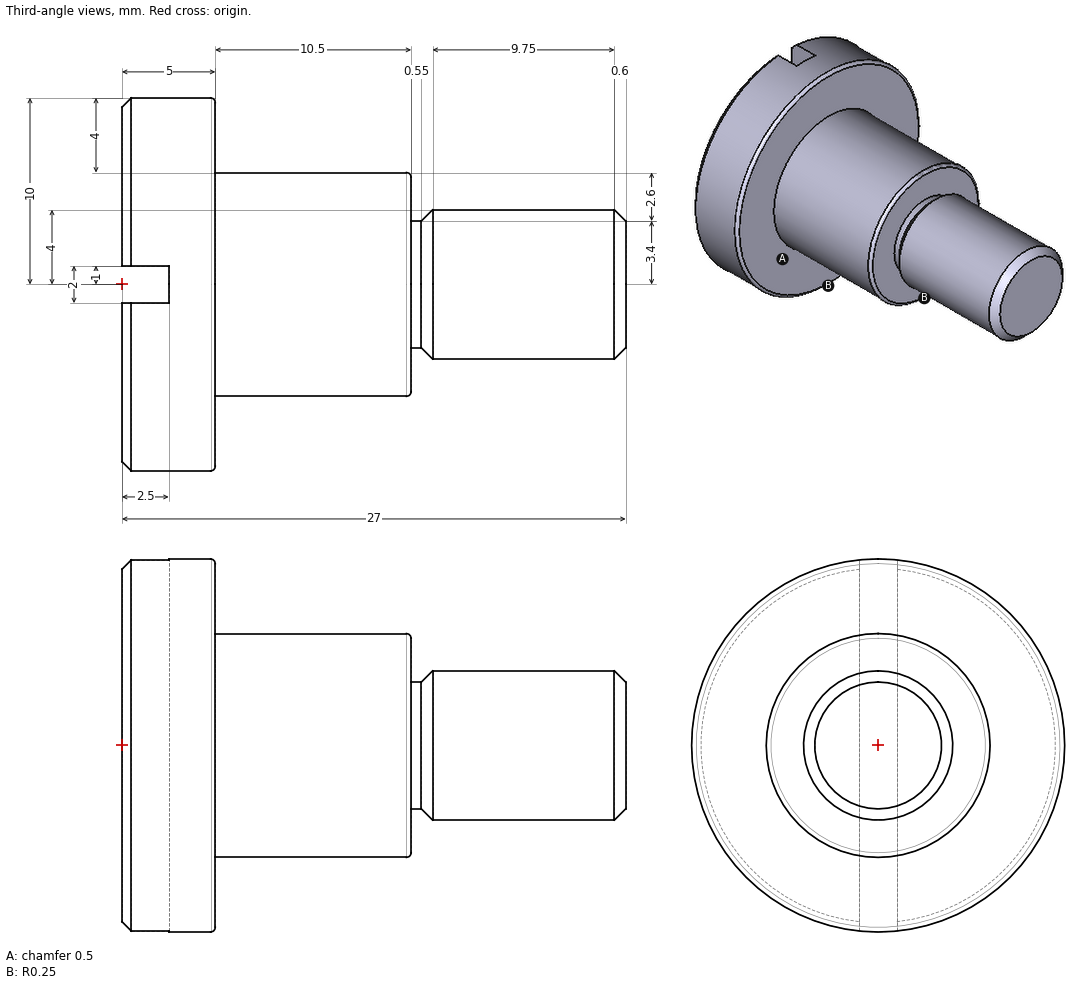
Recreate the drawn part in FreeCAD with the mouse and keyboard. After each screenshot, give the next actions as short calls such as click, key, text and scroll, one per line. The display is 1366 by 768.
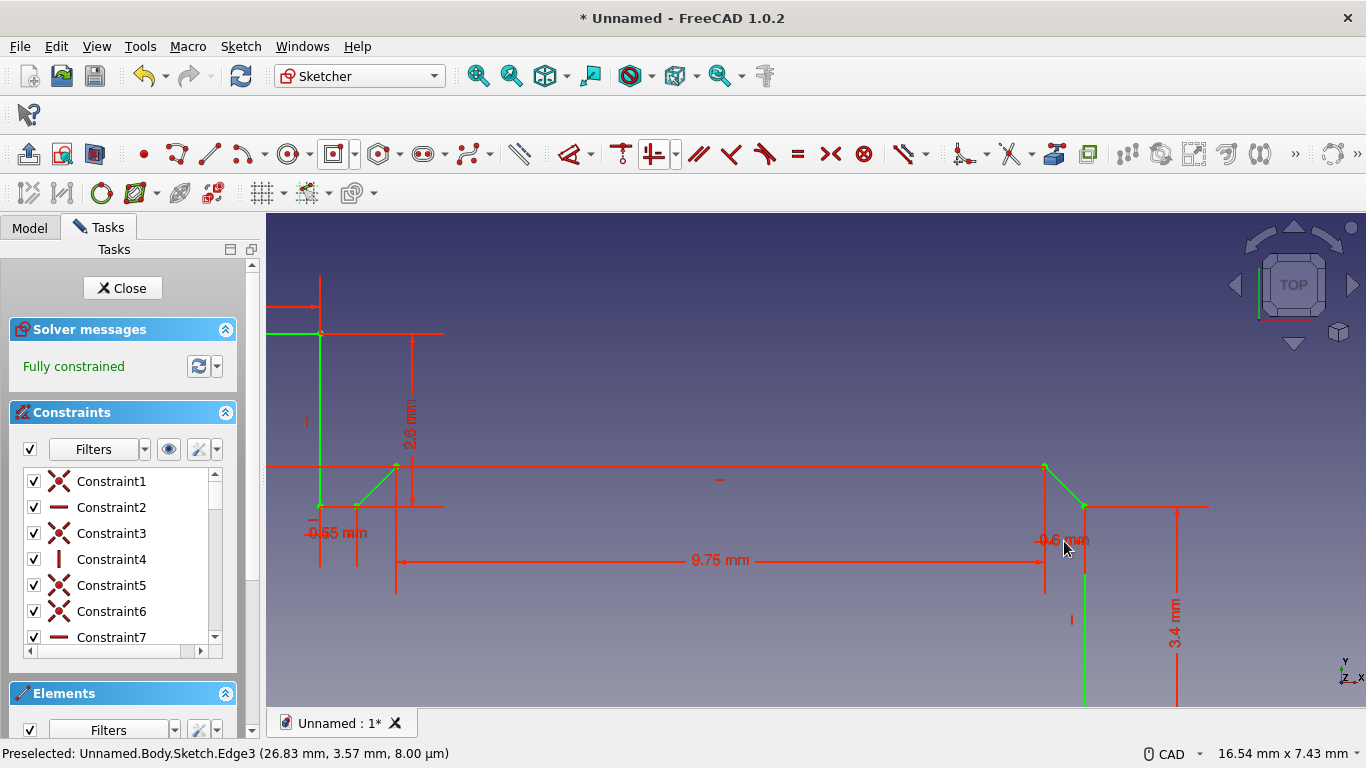
click(123, 288)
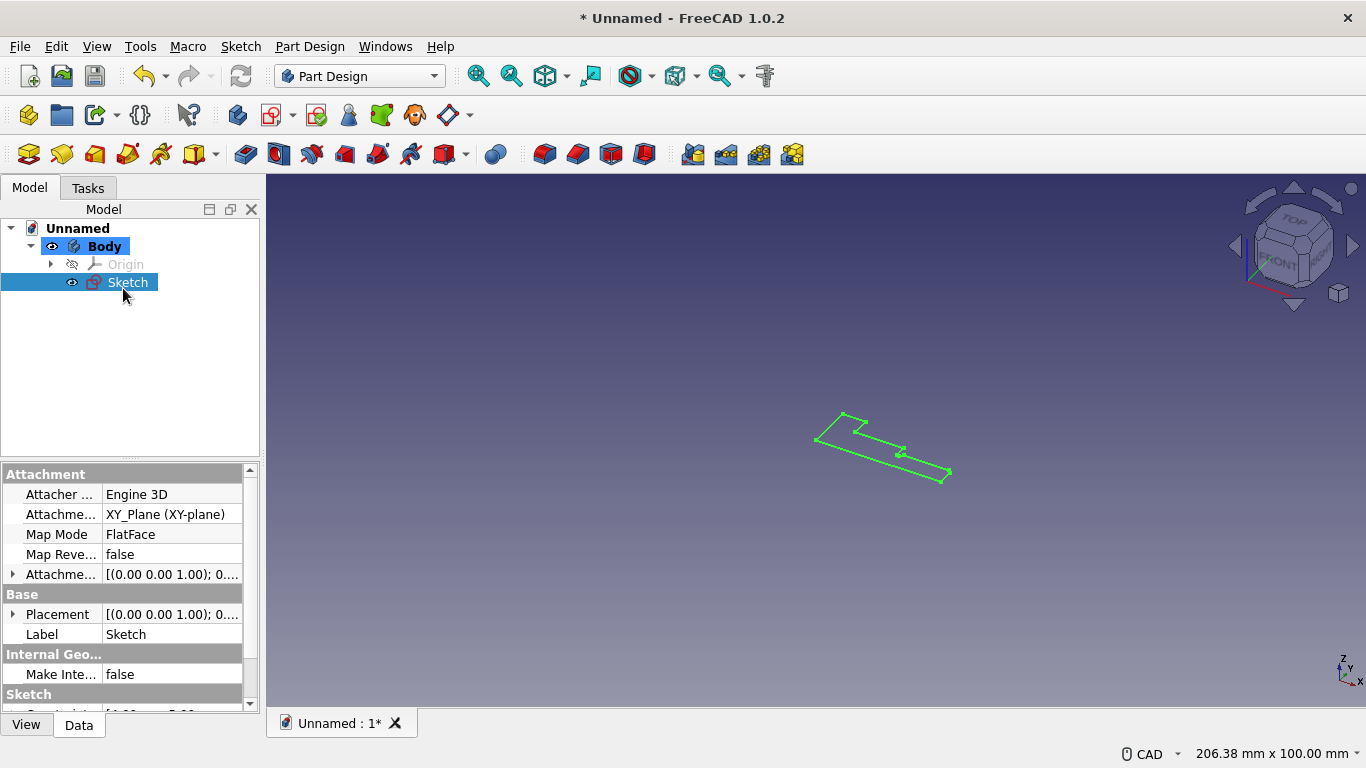
click(62, 154)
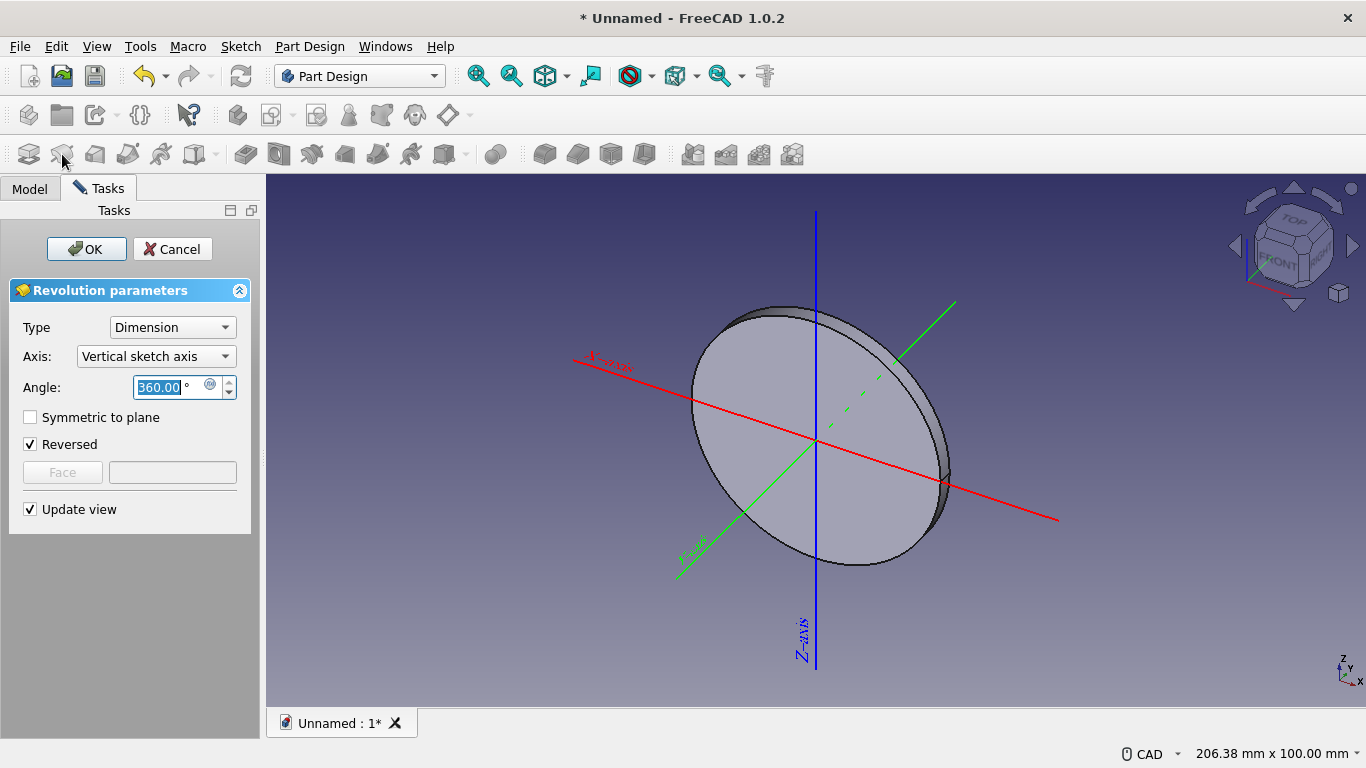
click(157, 356)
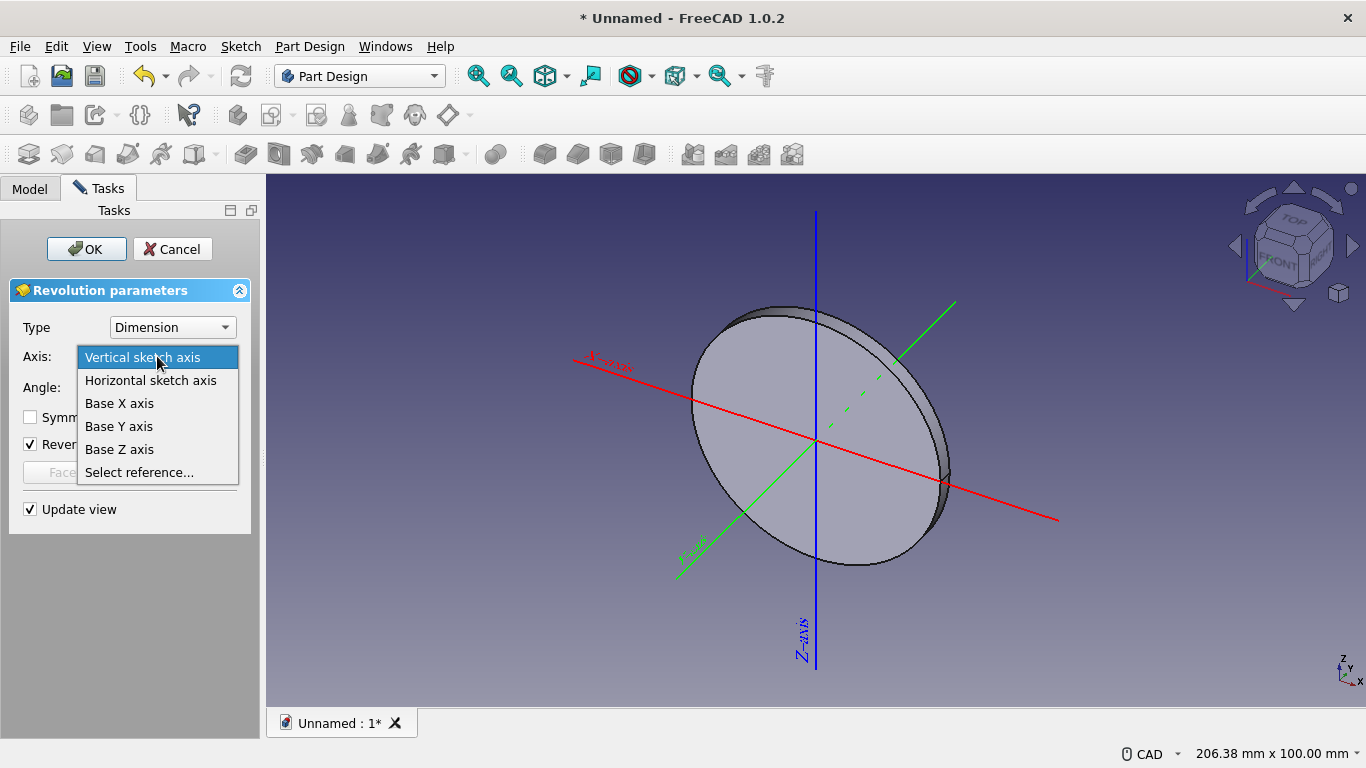
click(156, 380)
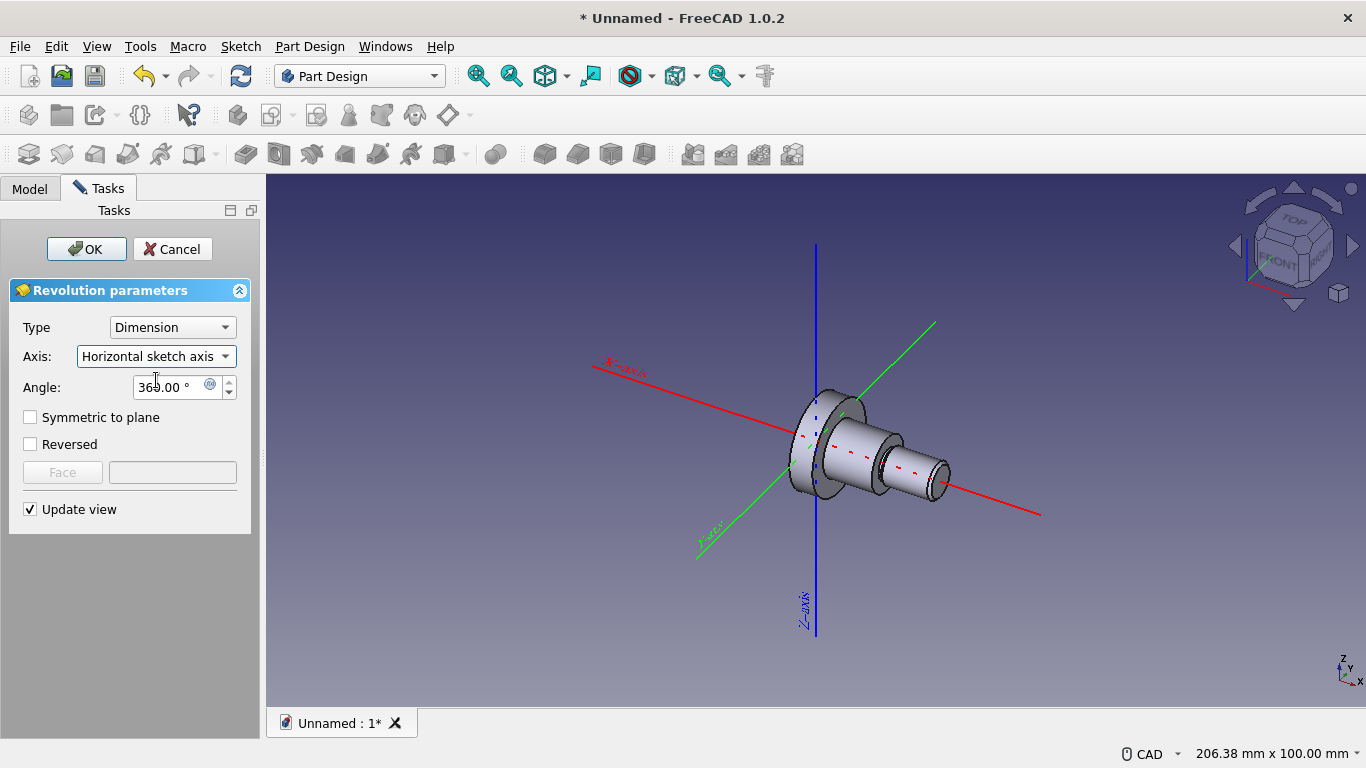
click(87, 249)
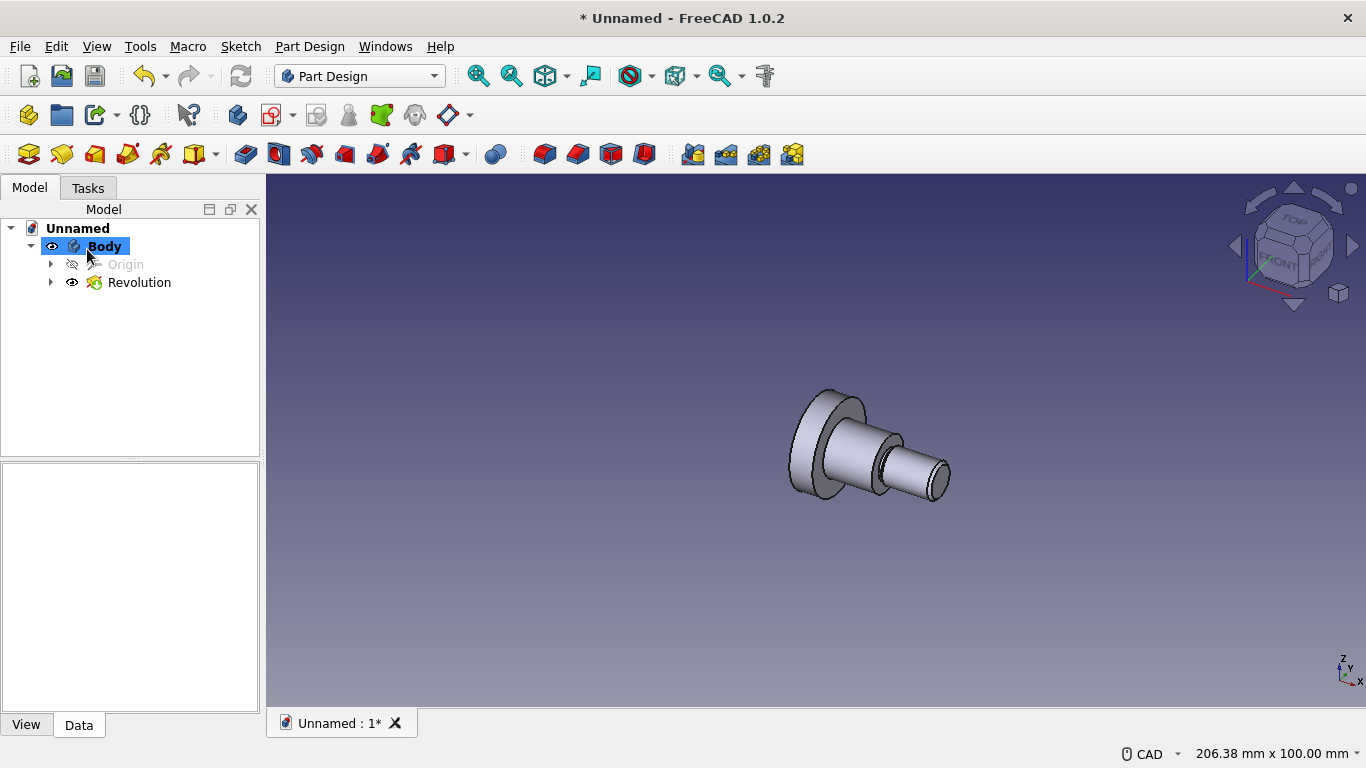
click(479, 76)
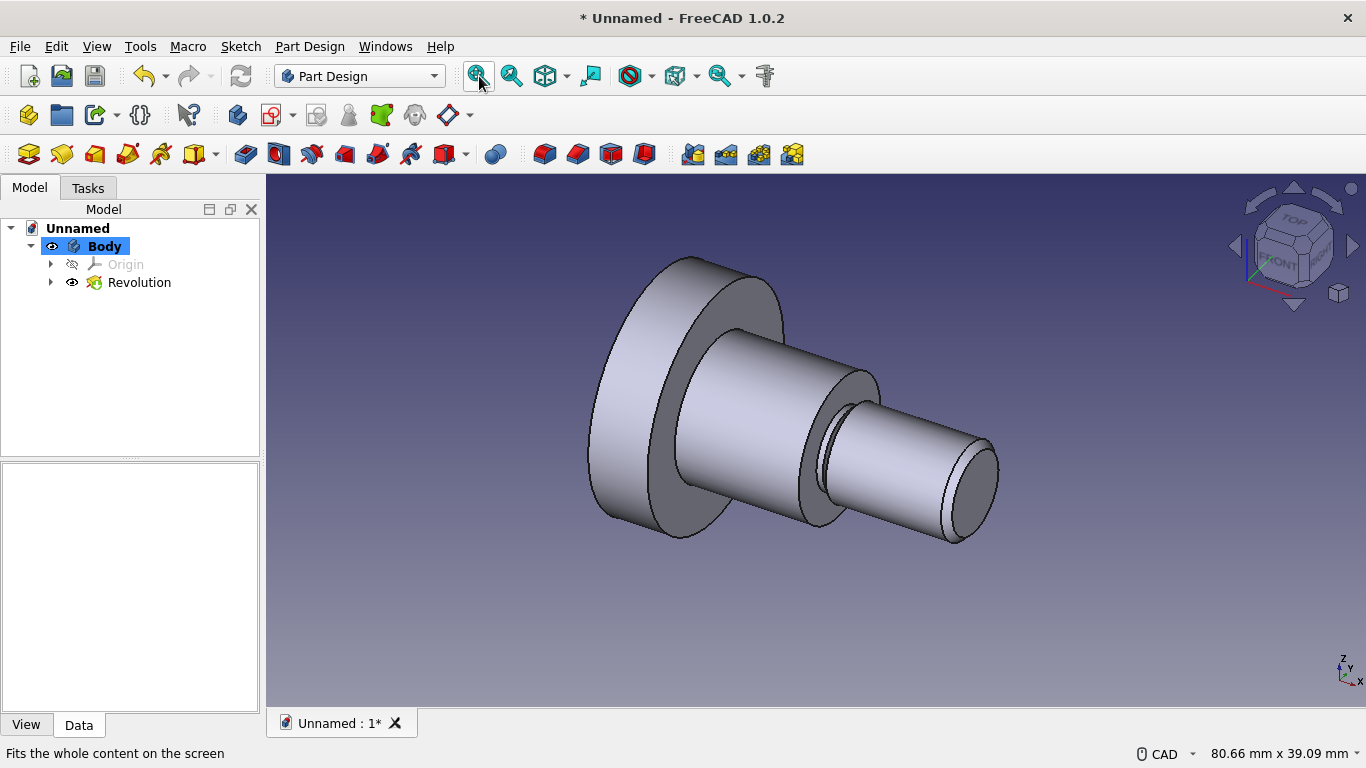
key(0)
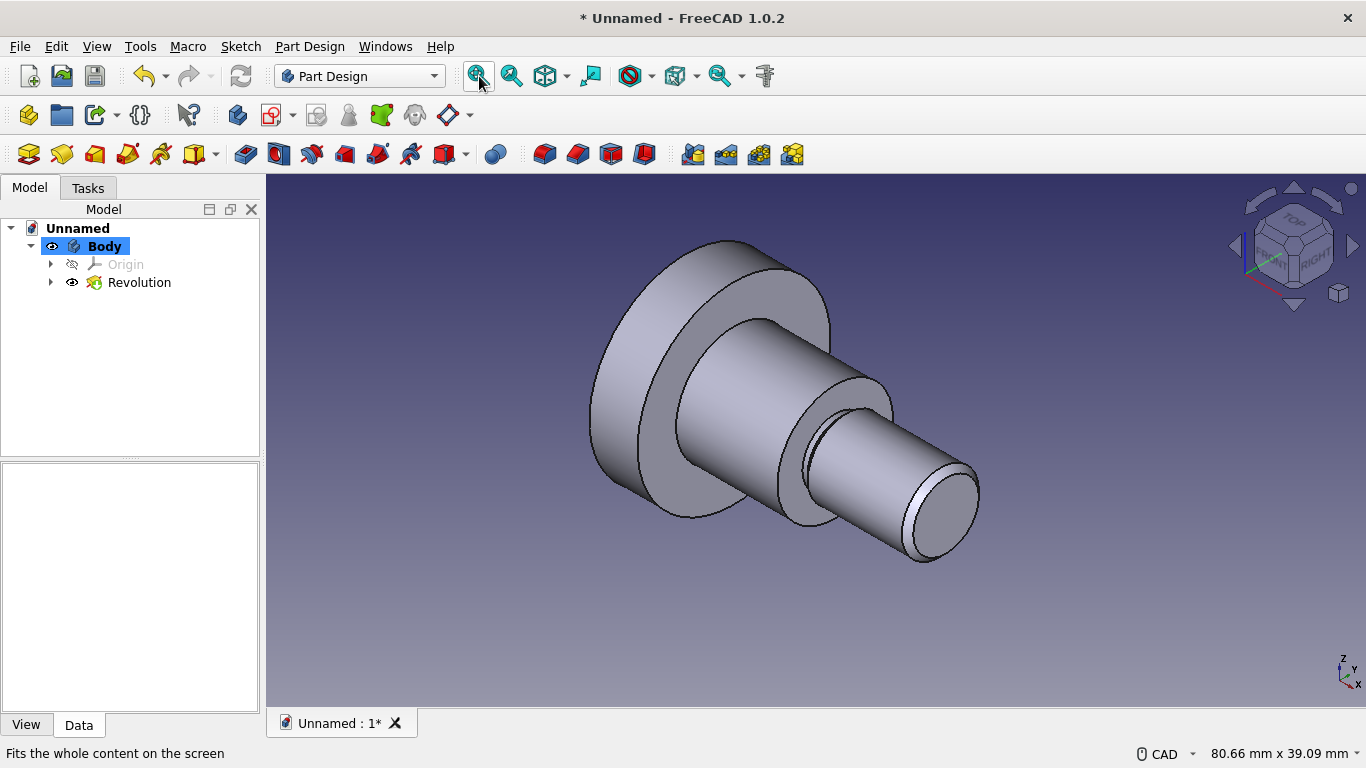
key(2)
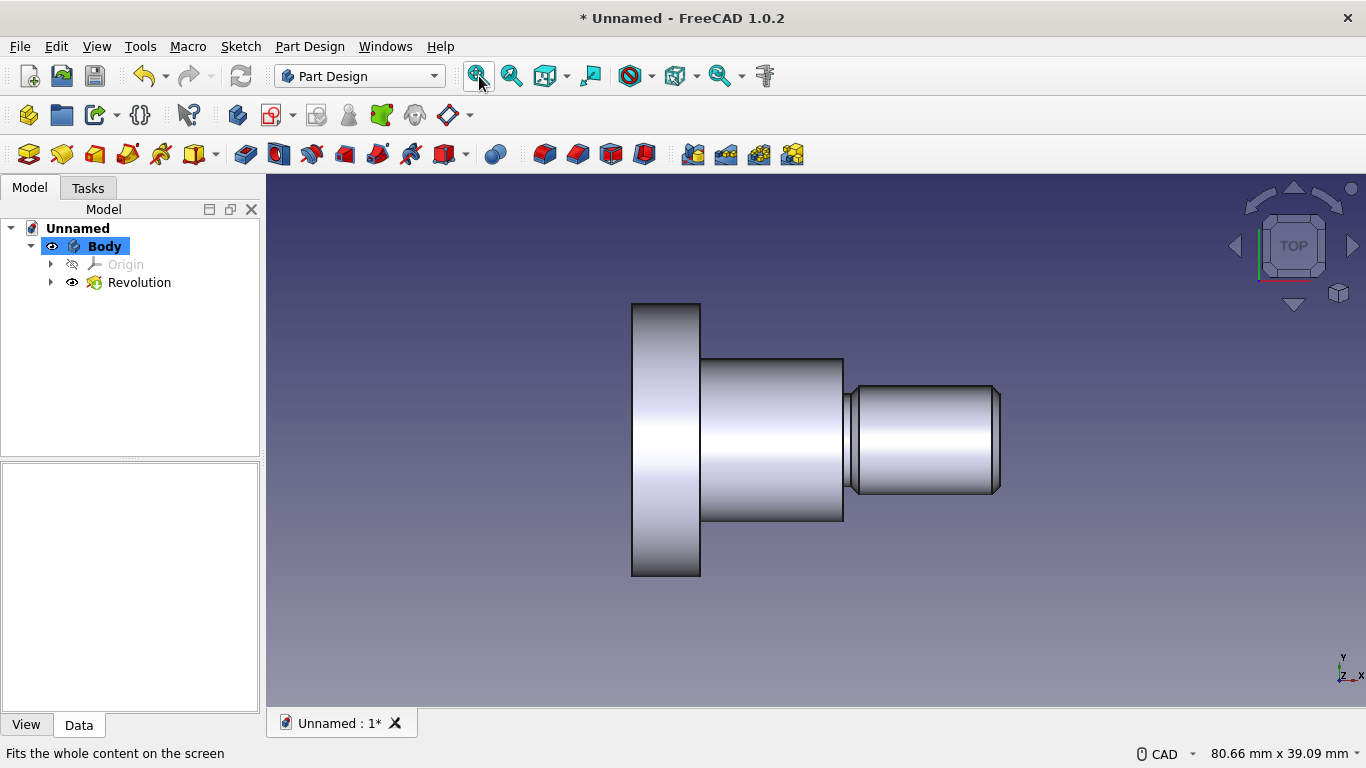
click(632, 550)